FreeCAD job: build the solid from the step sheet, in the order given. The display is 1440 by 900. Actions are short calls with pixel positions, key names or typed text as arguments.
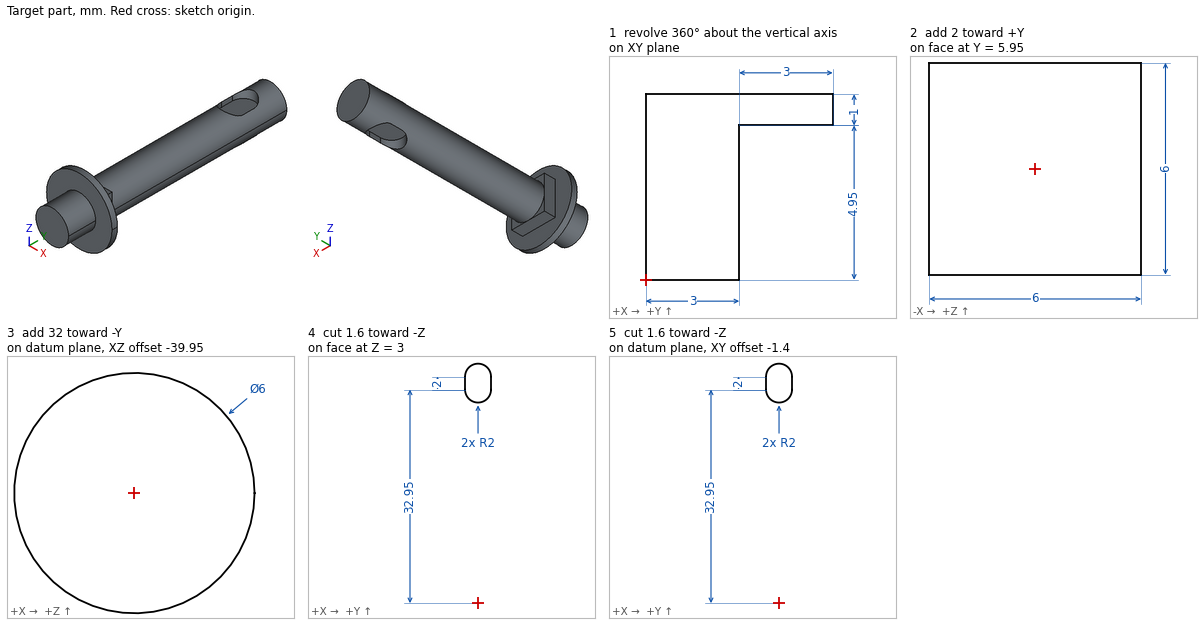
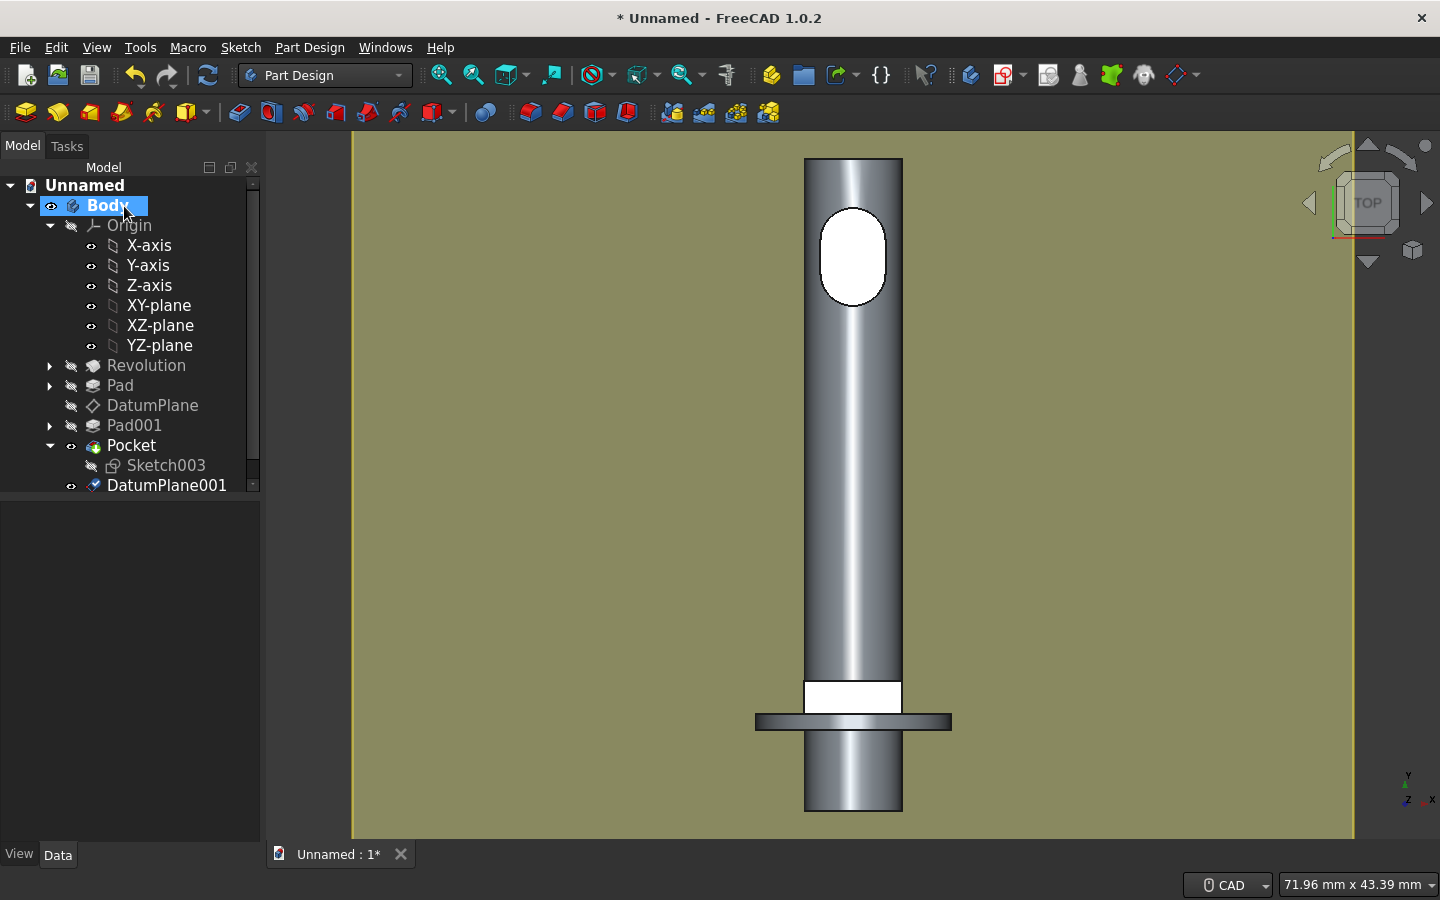
click(116, 486)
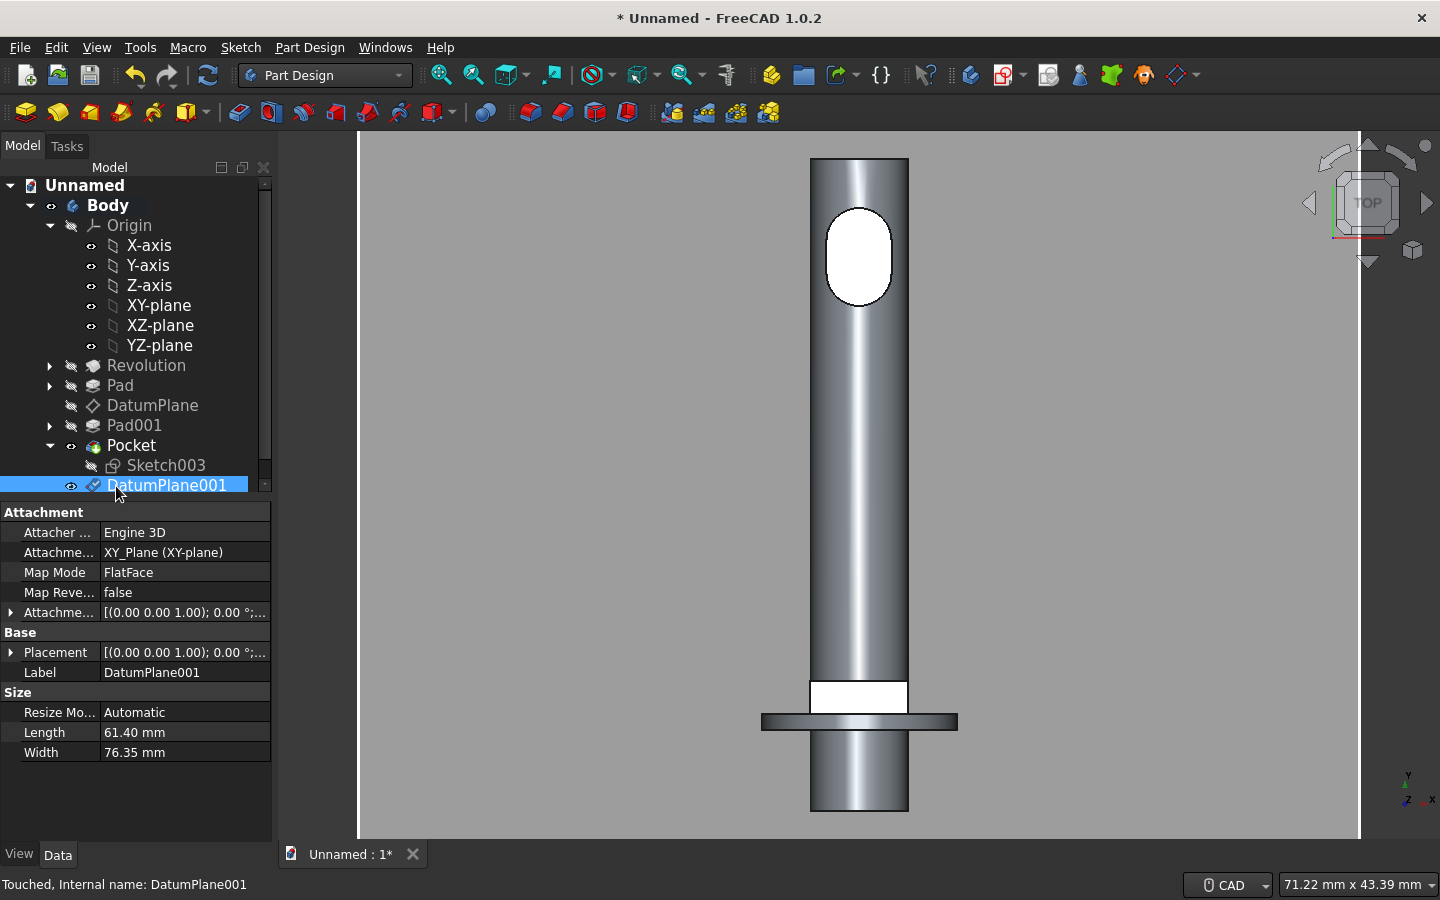
click(1004, 76)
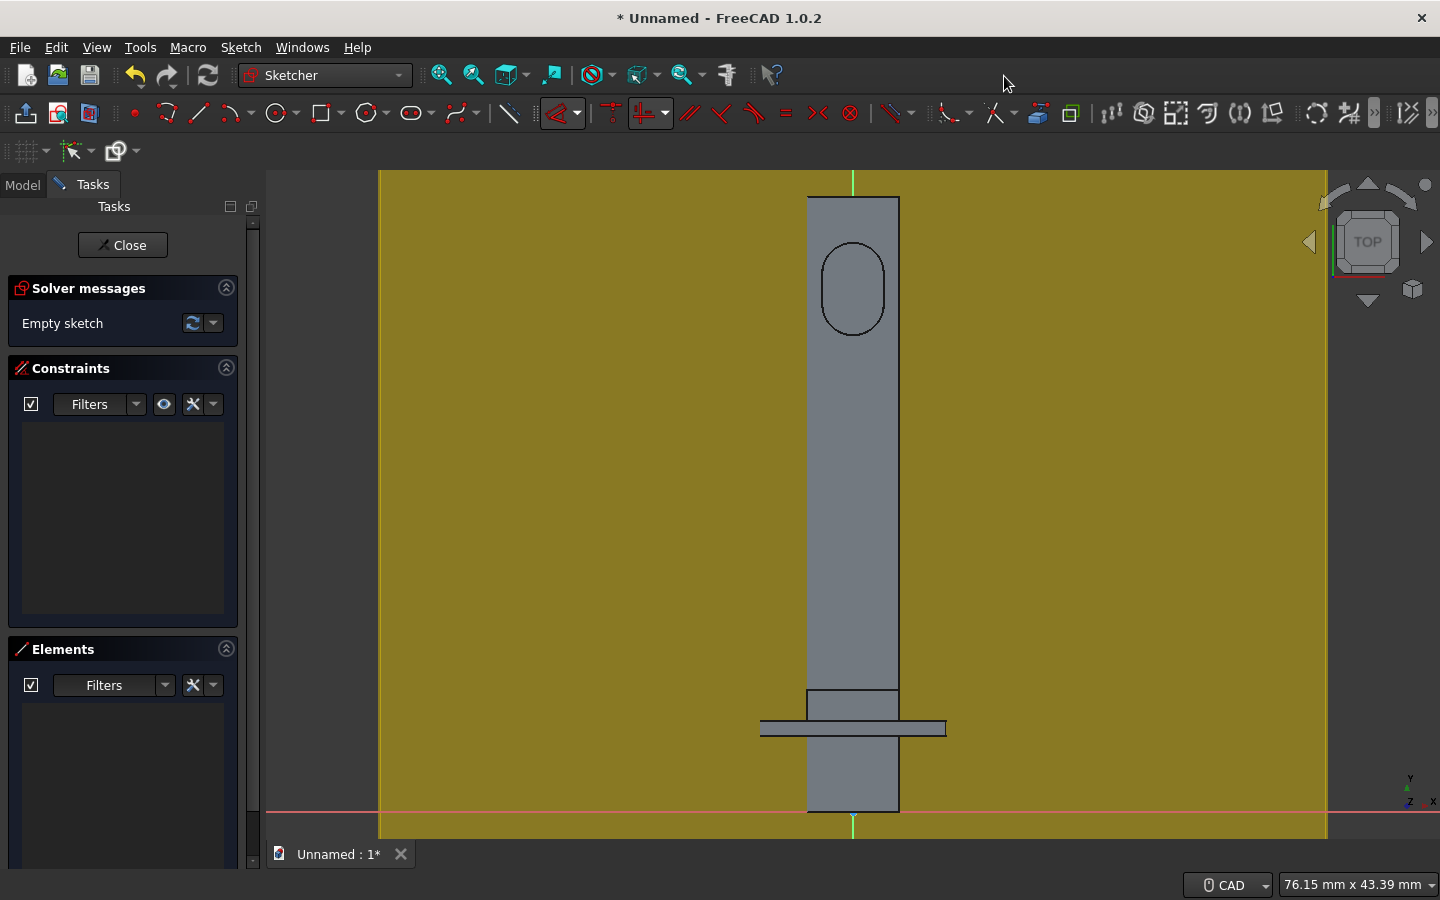
click(90, 114)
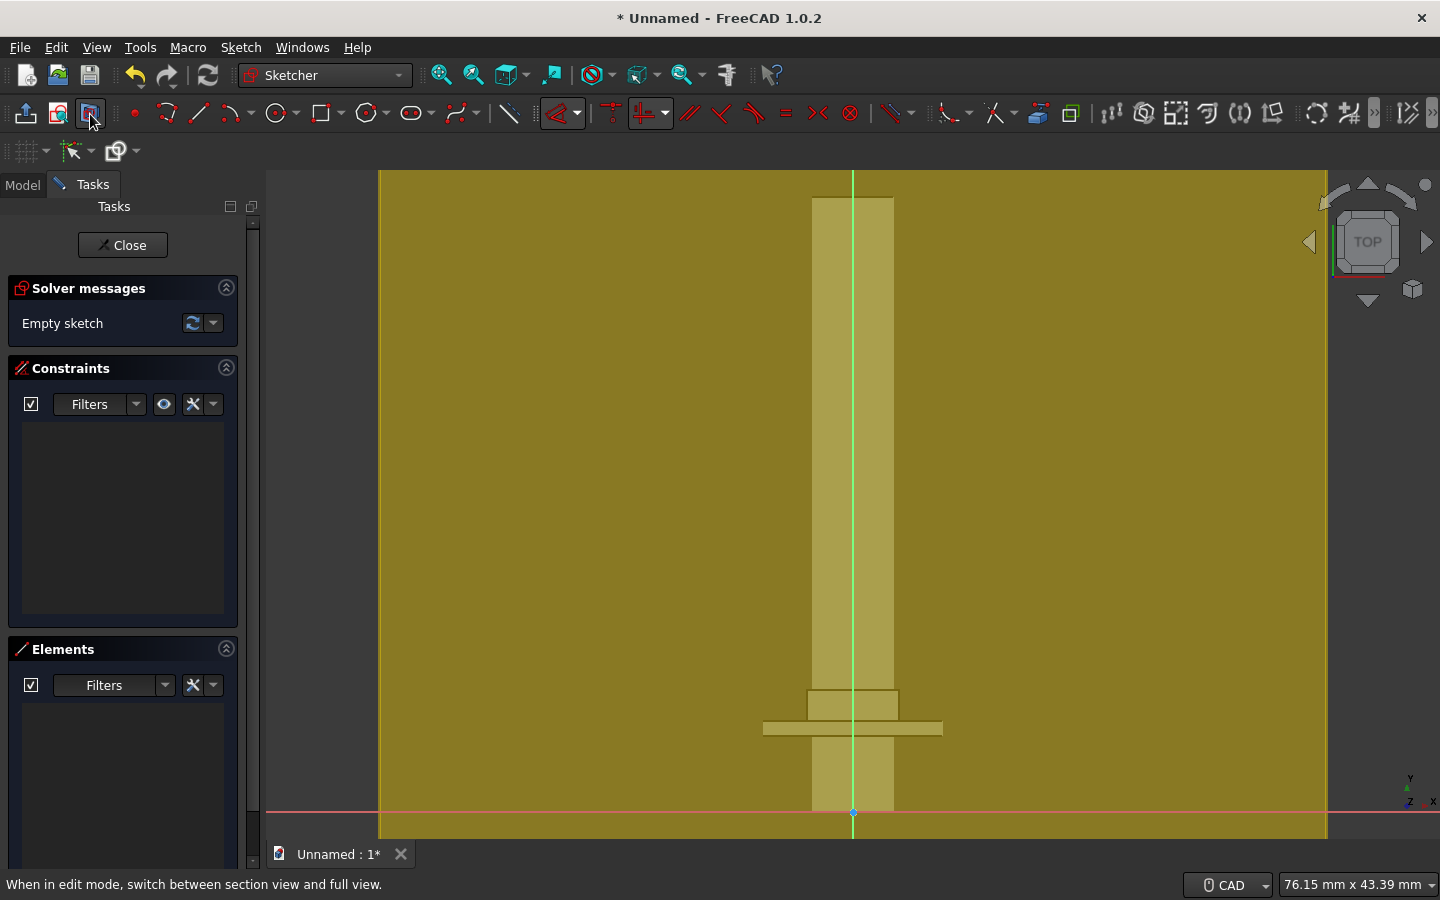
scroll(870, 235, up, 8)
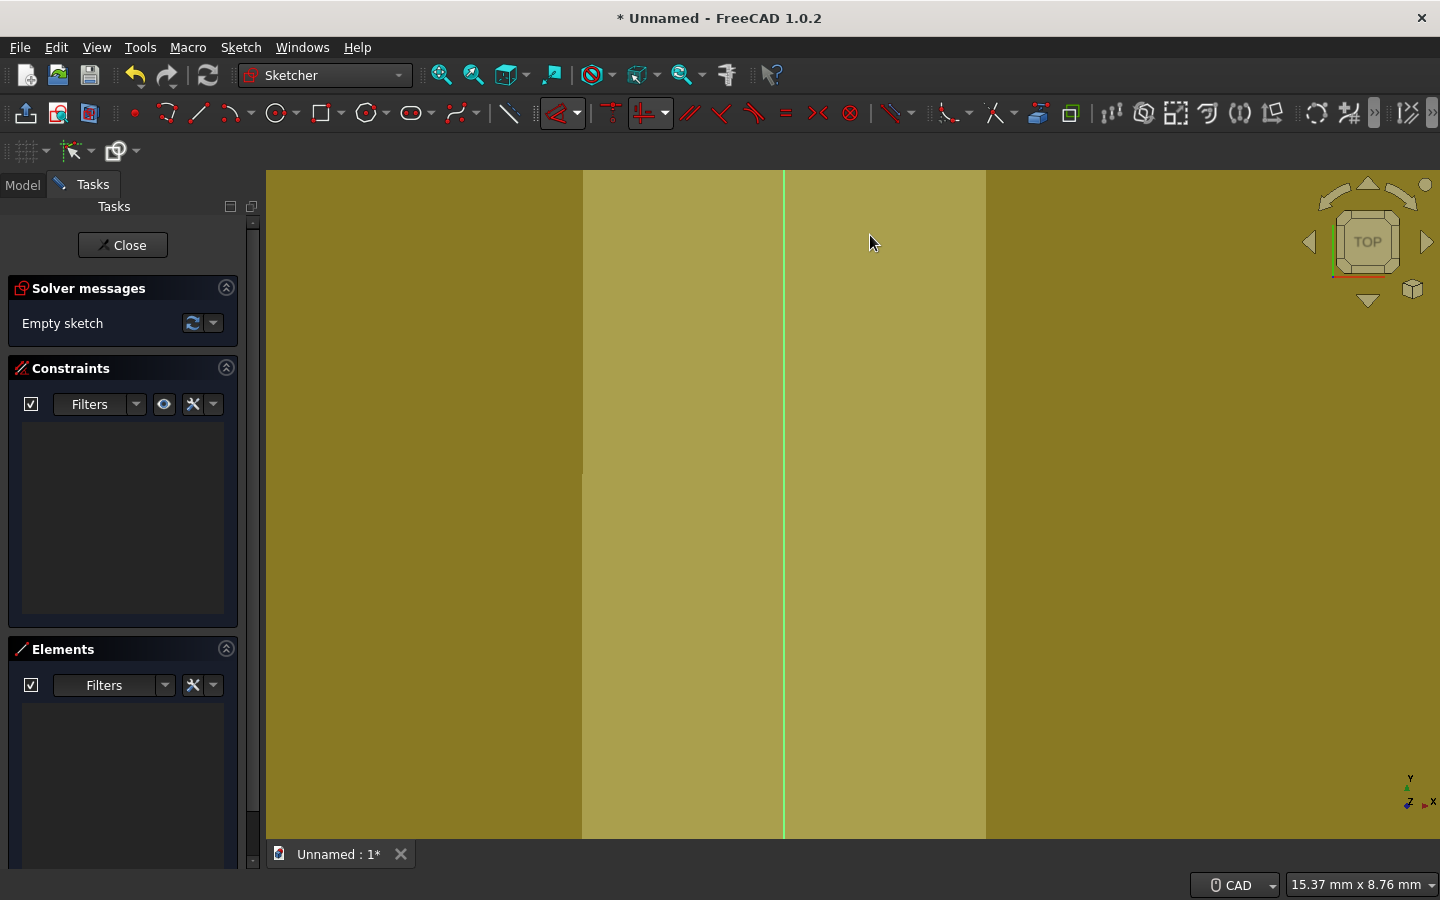
click(412, 114)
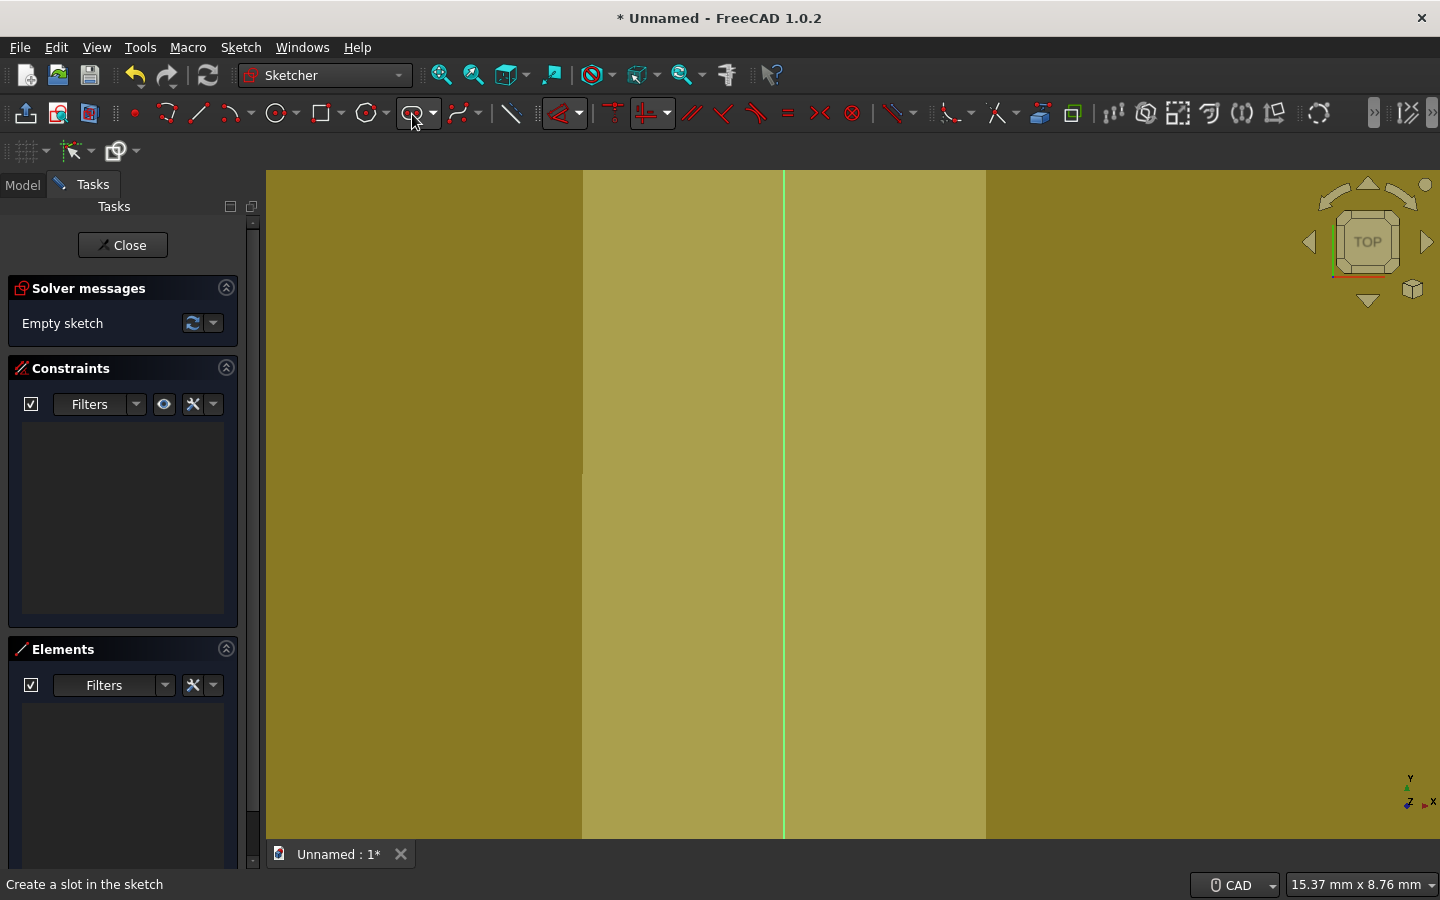
click(784, 579)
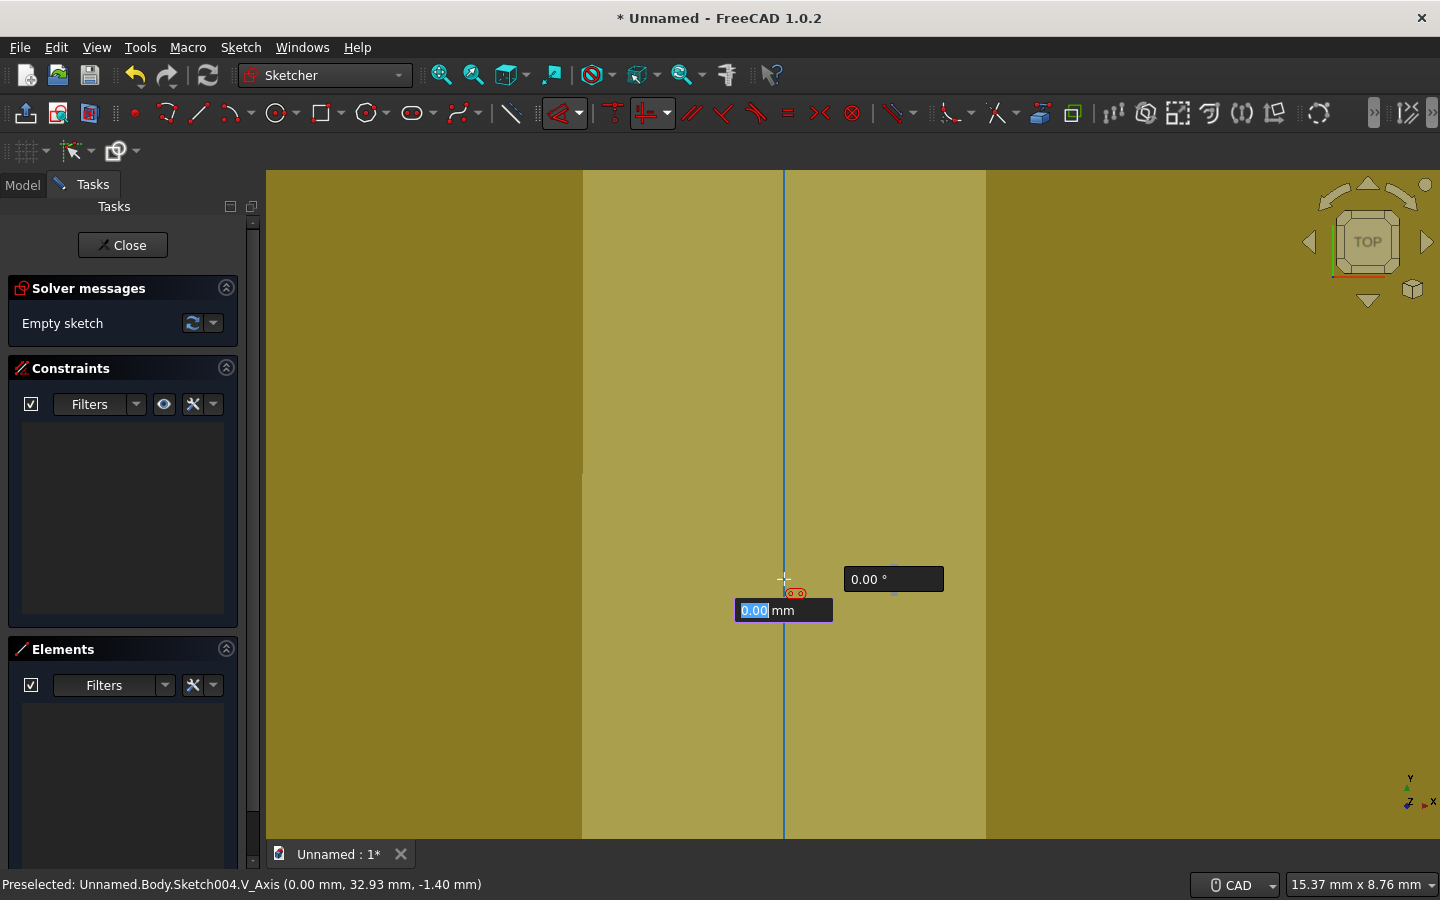
click(793, 426)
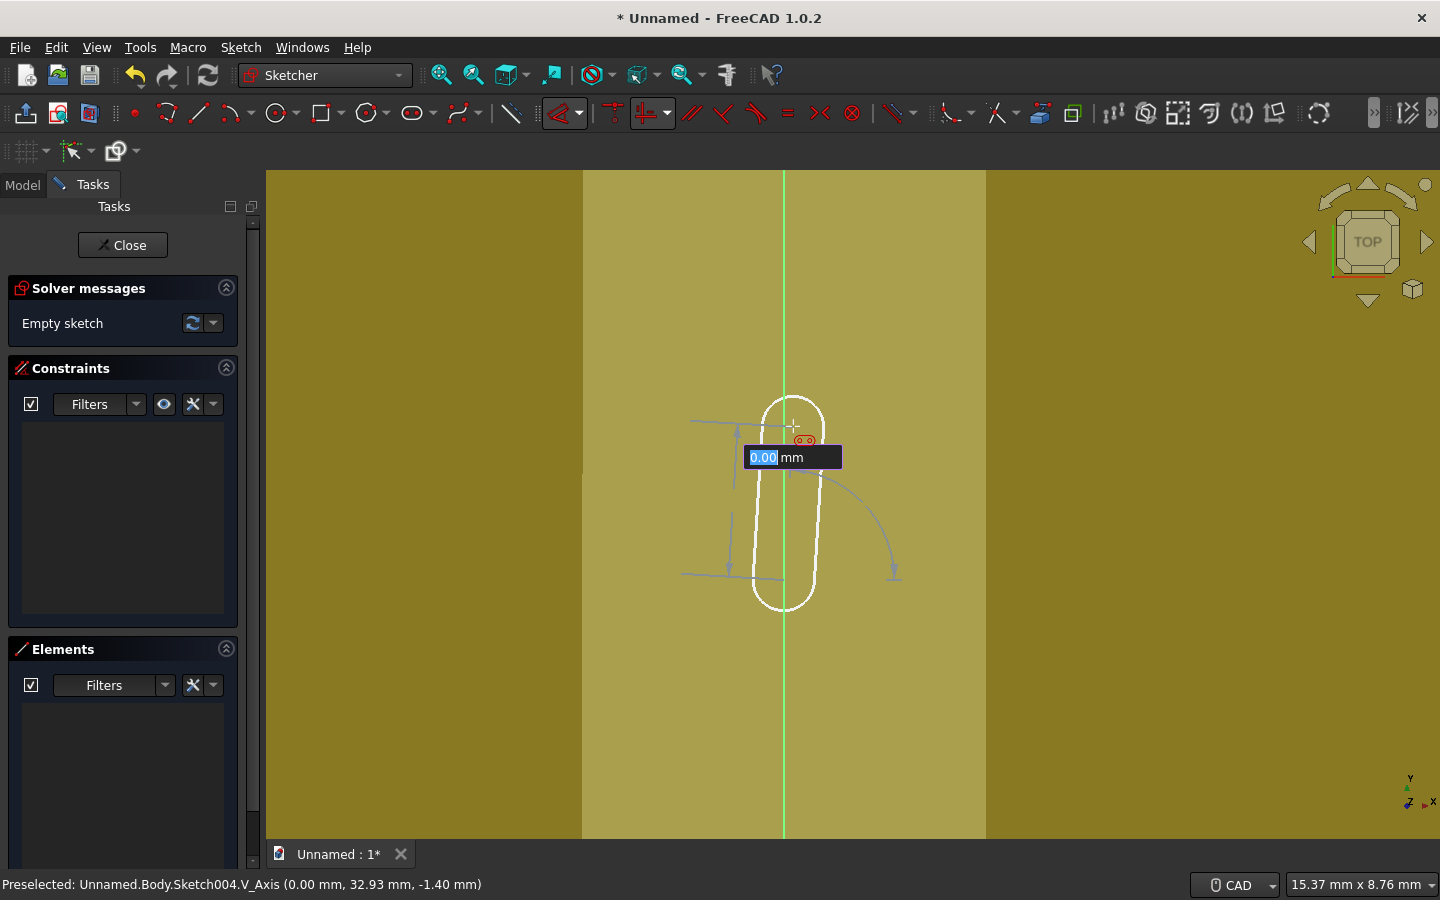
click(631, 502)
key(Escape)